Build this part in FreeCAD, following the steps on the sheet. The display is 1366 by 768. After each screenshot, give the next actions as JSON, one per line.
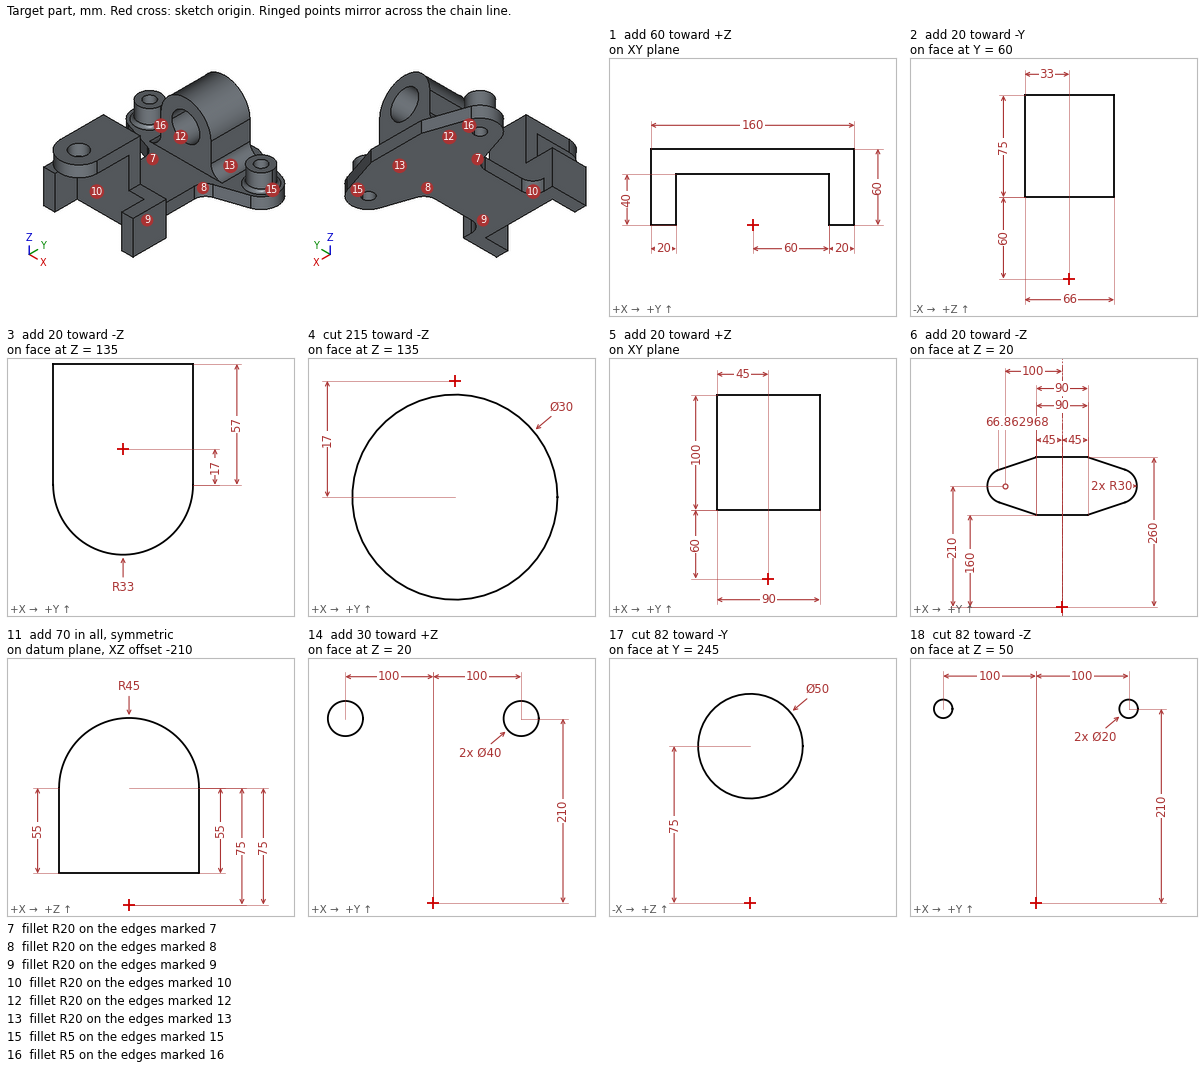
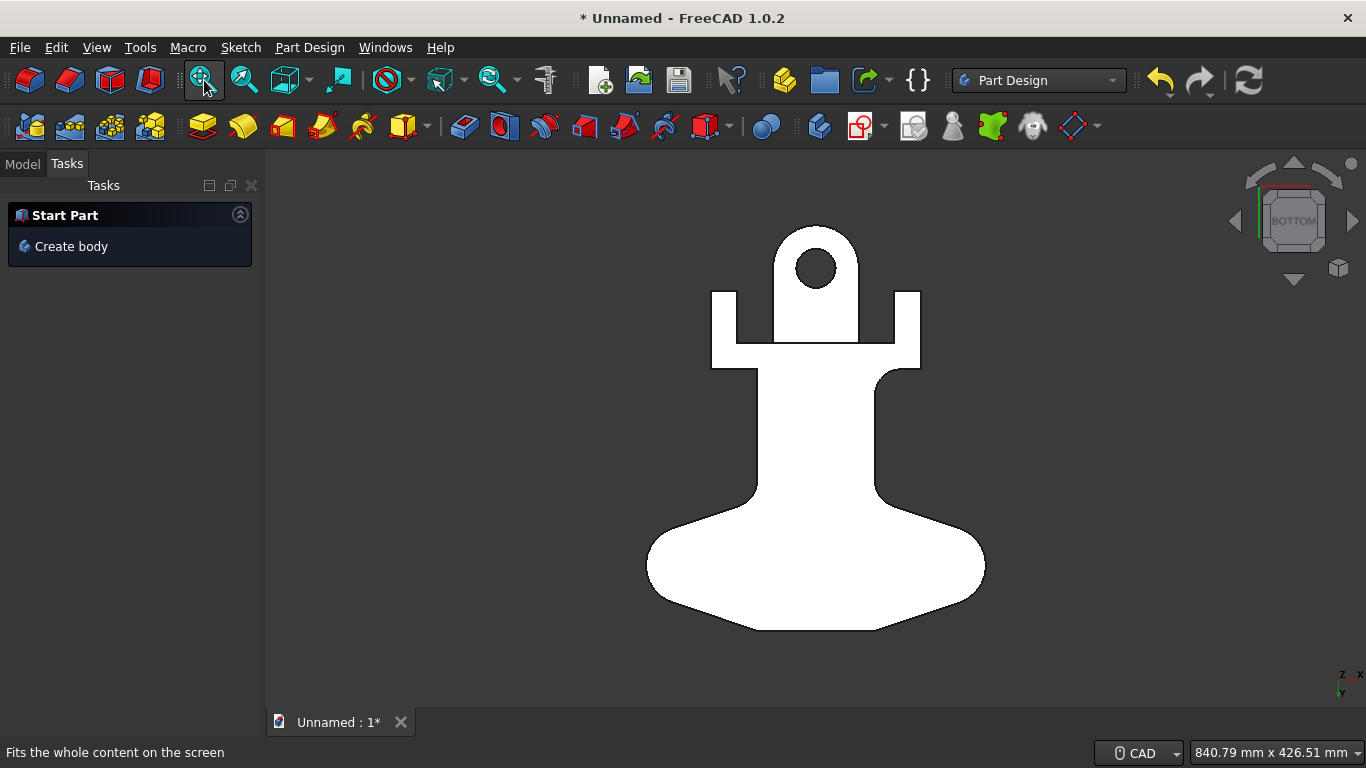
{"action": "key", "text": "4"}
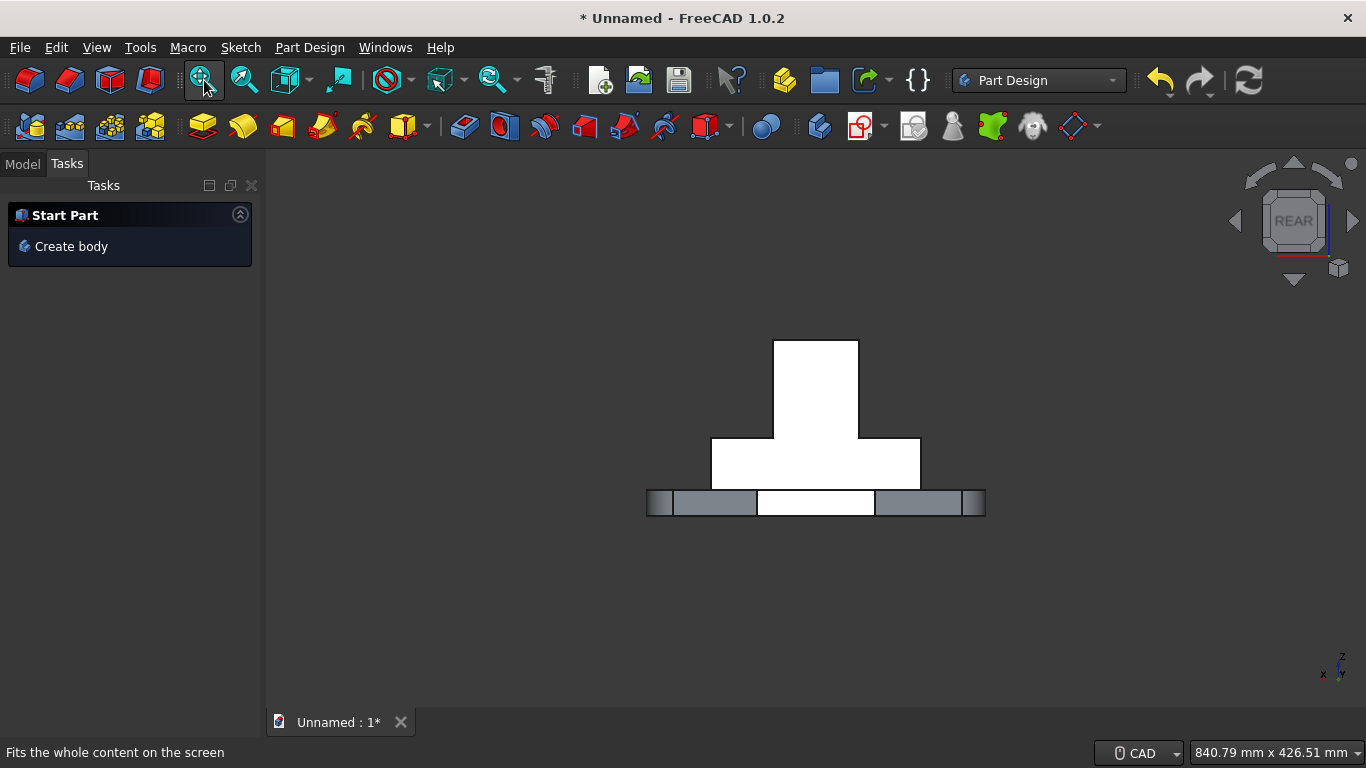
{"action": "key", "text": "v f"}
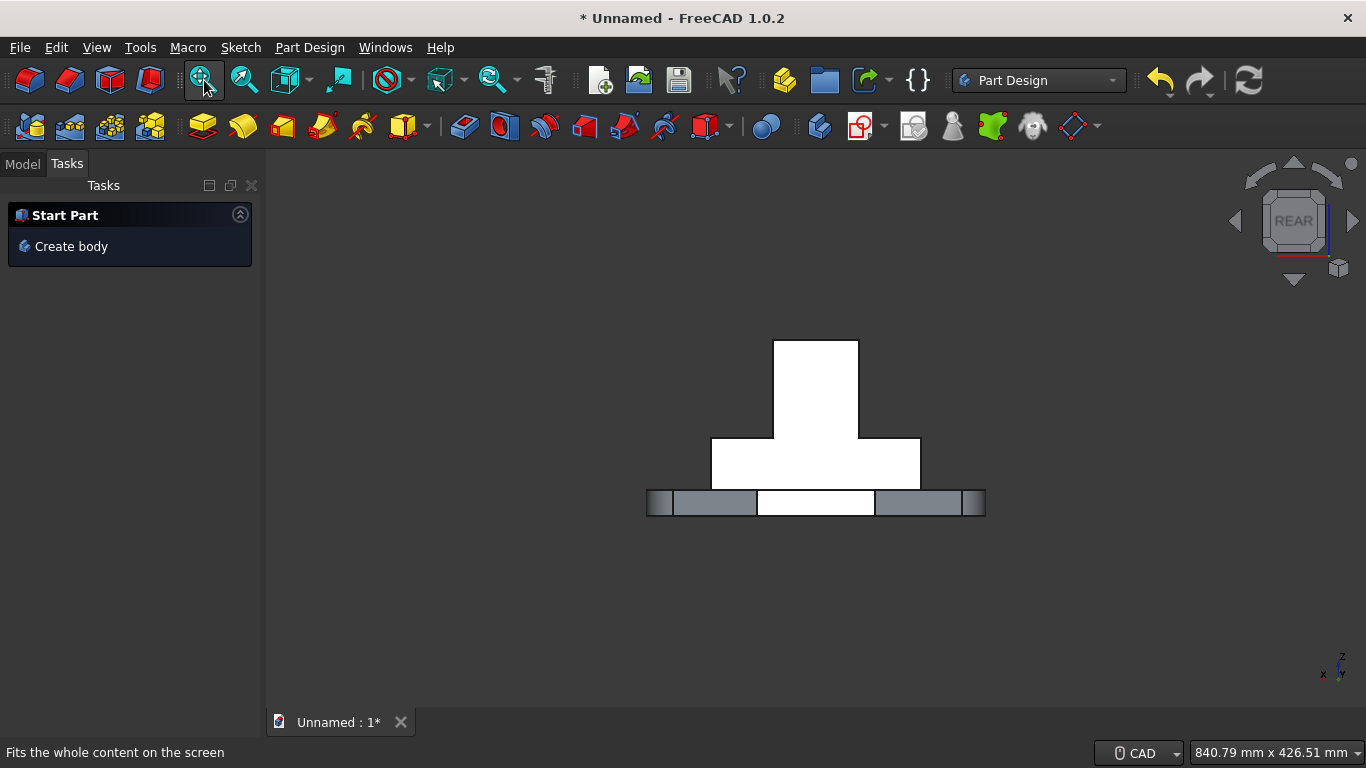
{"action": "key", "text": "6"}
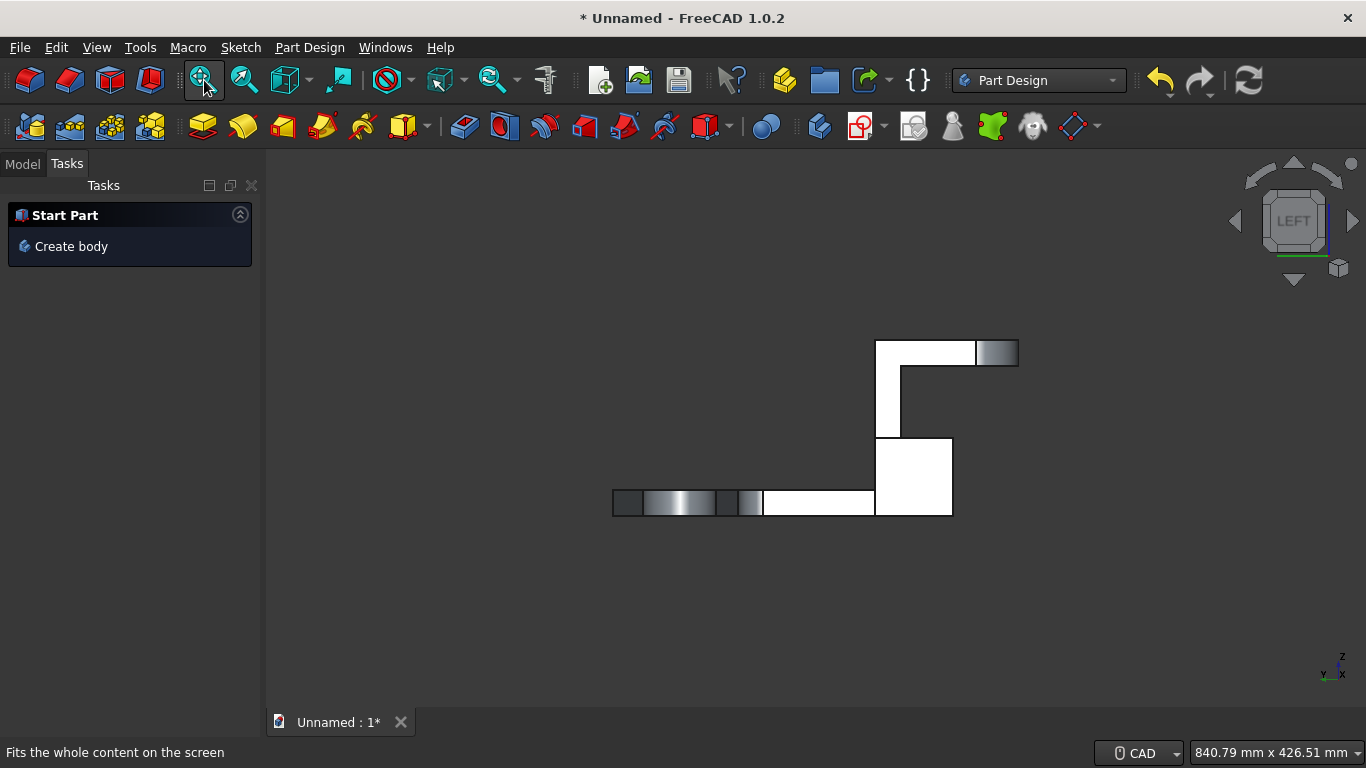
{"action": "key", "text": "v f"}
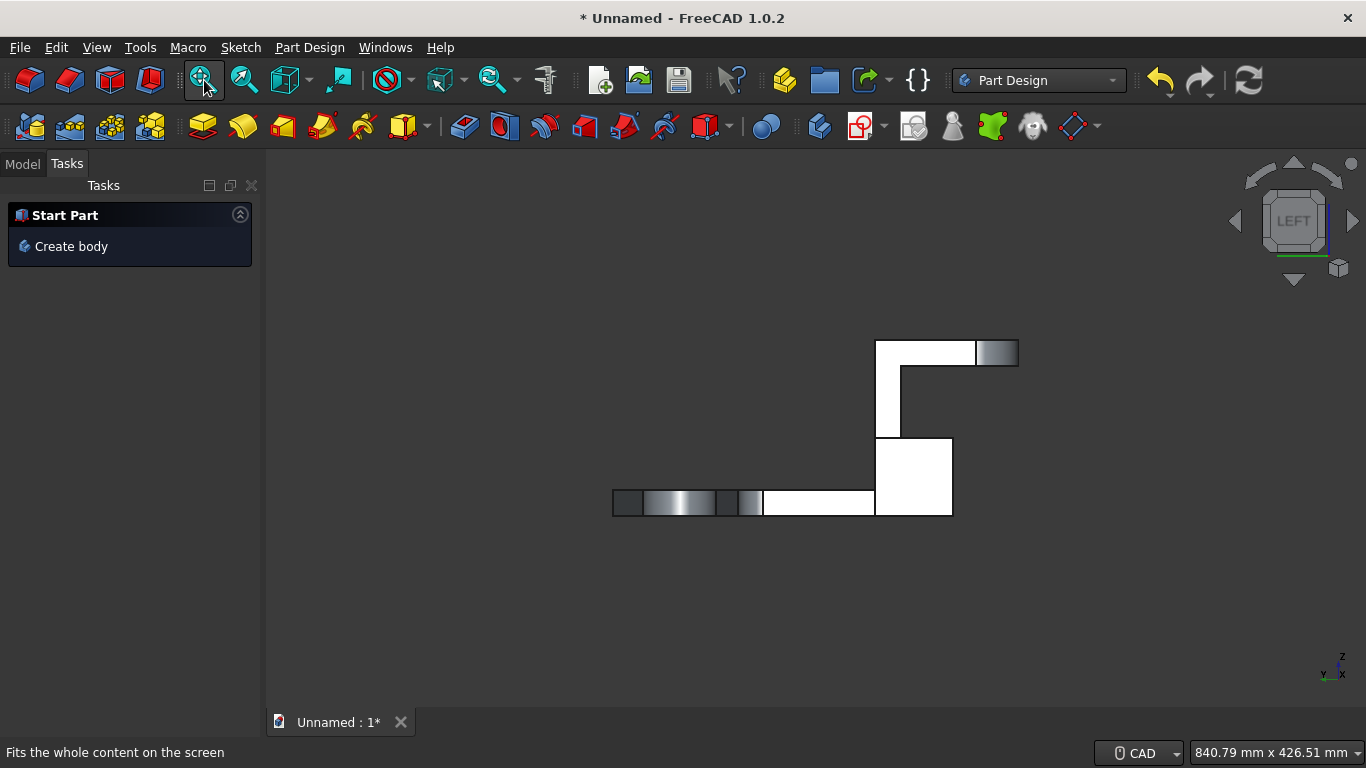
{"action": "key", "text": "v 3"}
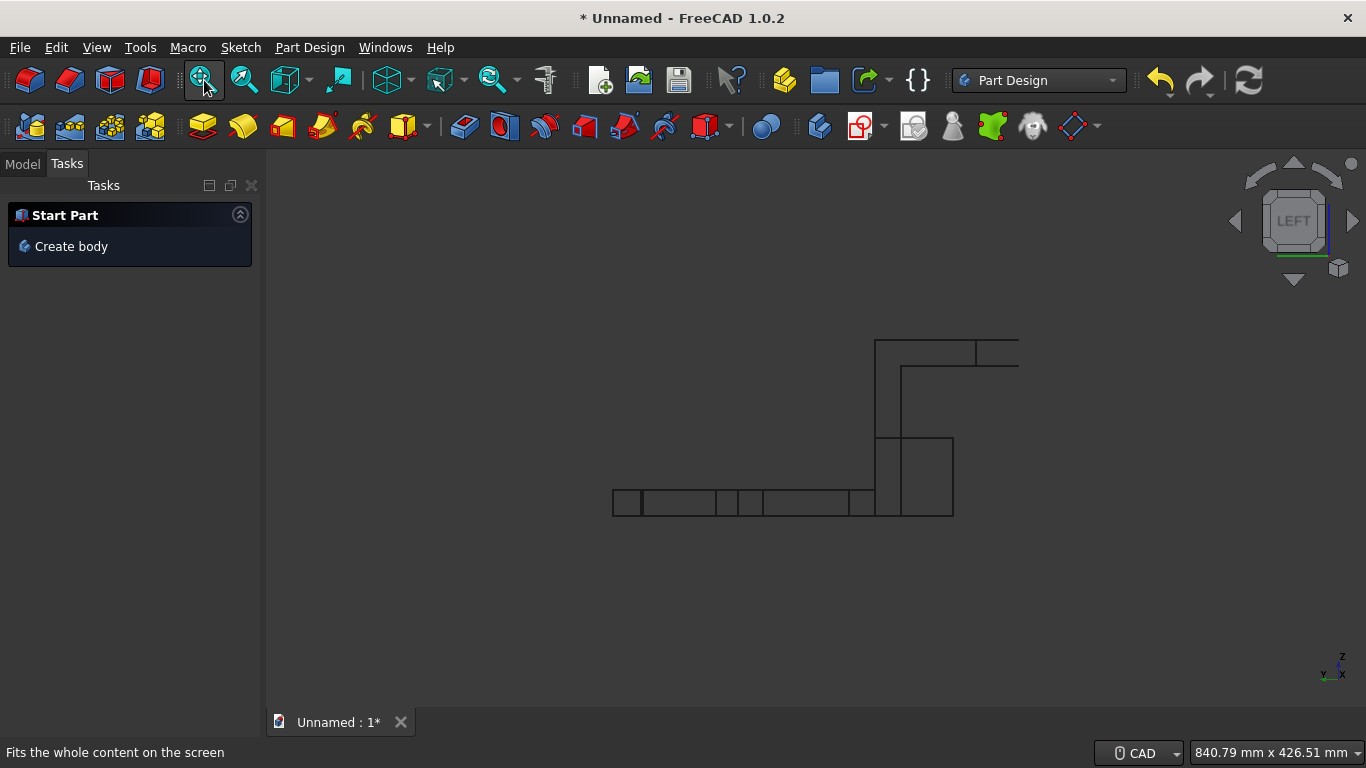
{"action": "key", "text": "0"}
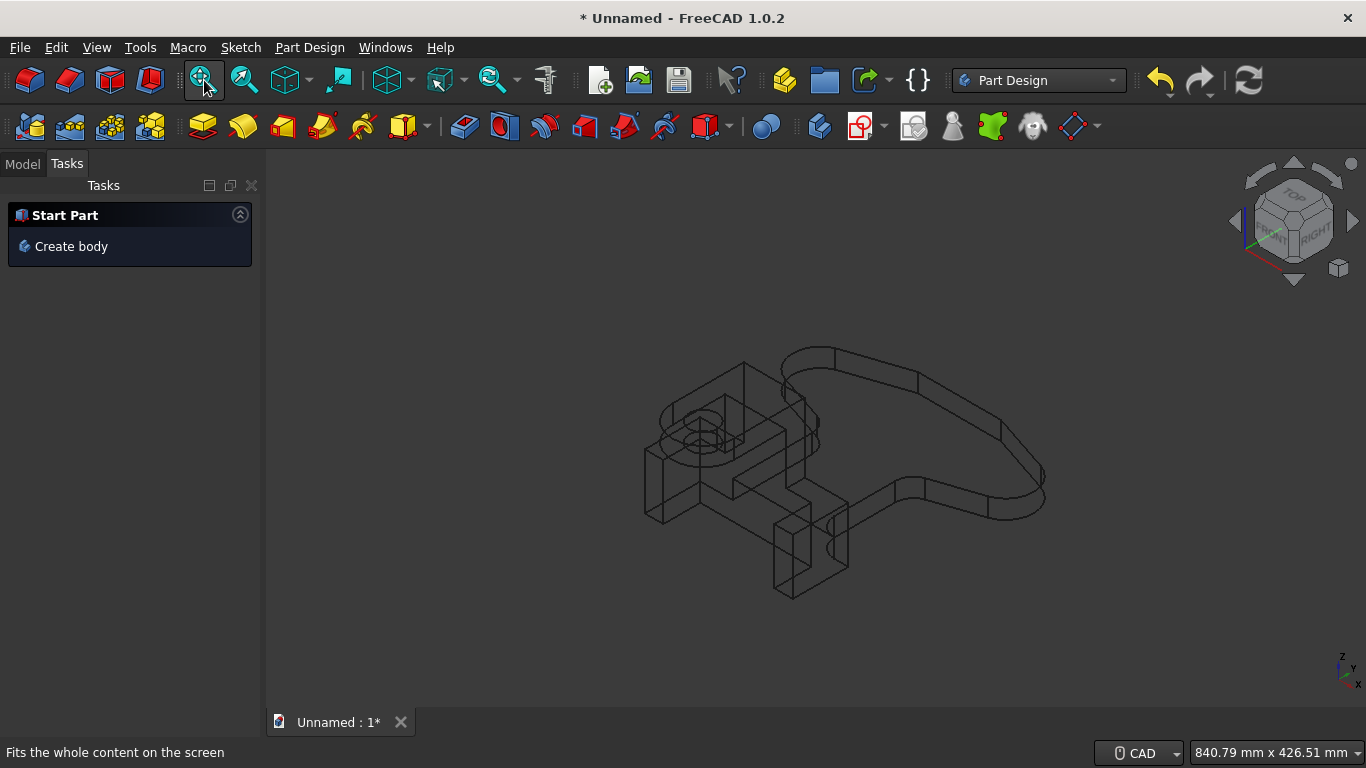
{"action": "left_click", "coordinate": [733, 488]}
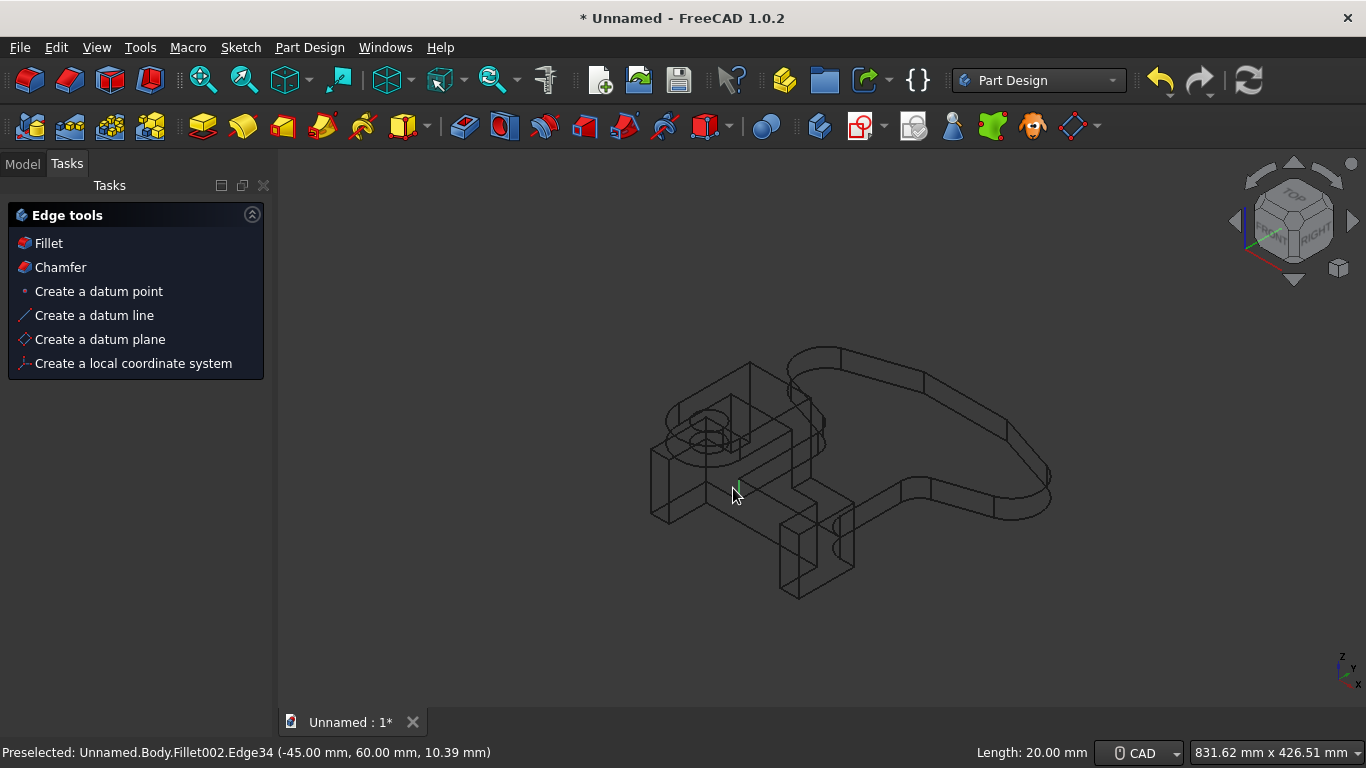
{"action": "key", "text": "v 1"}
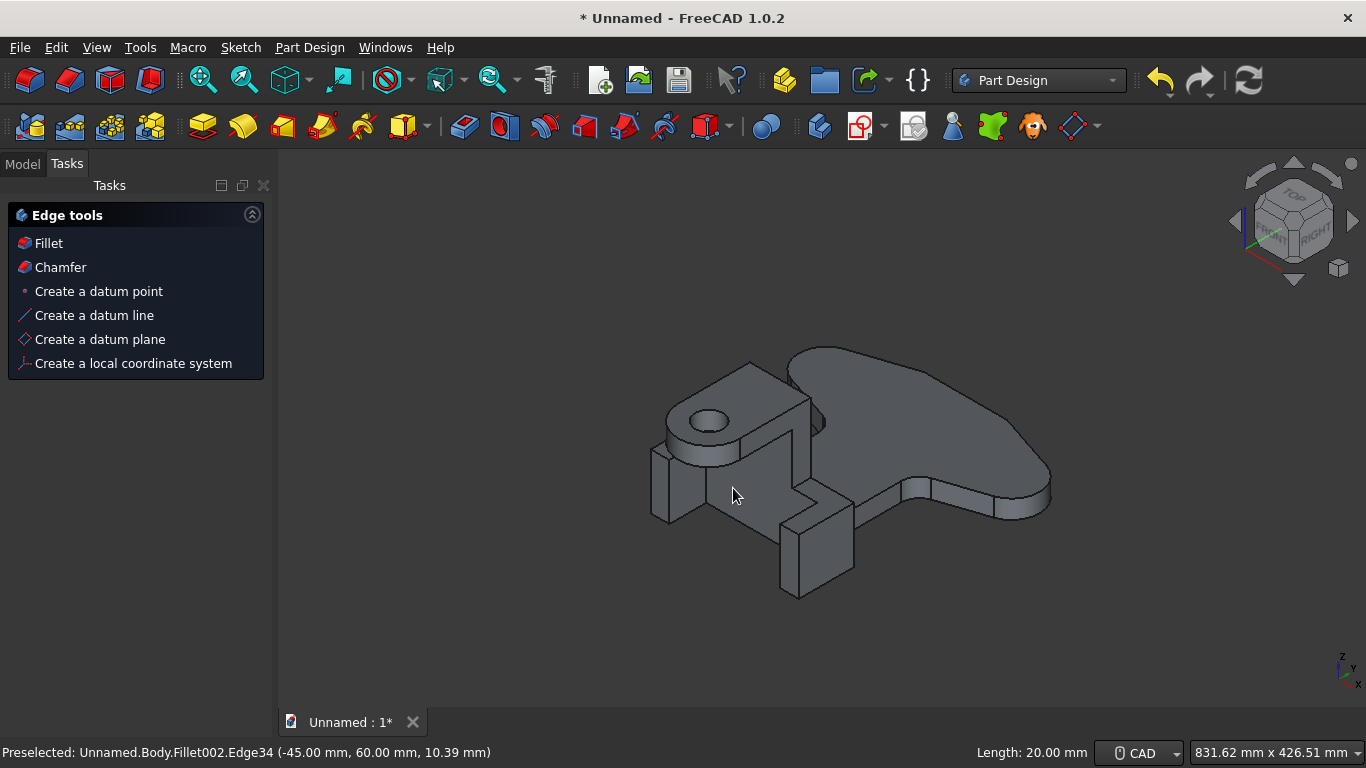
{"action": "left_click", "coordinate": [30, 80]}